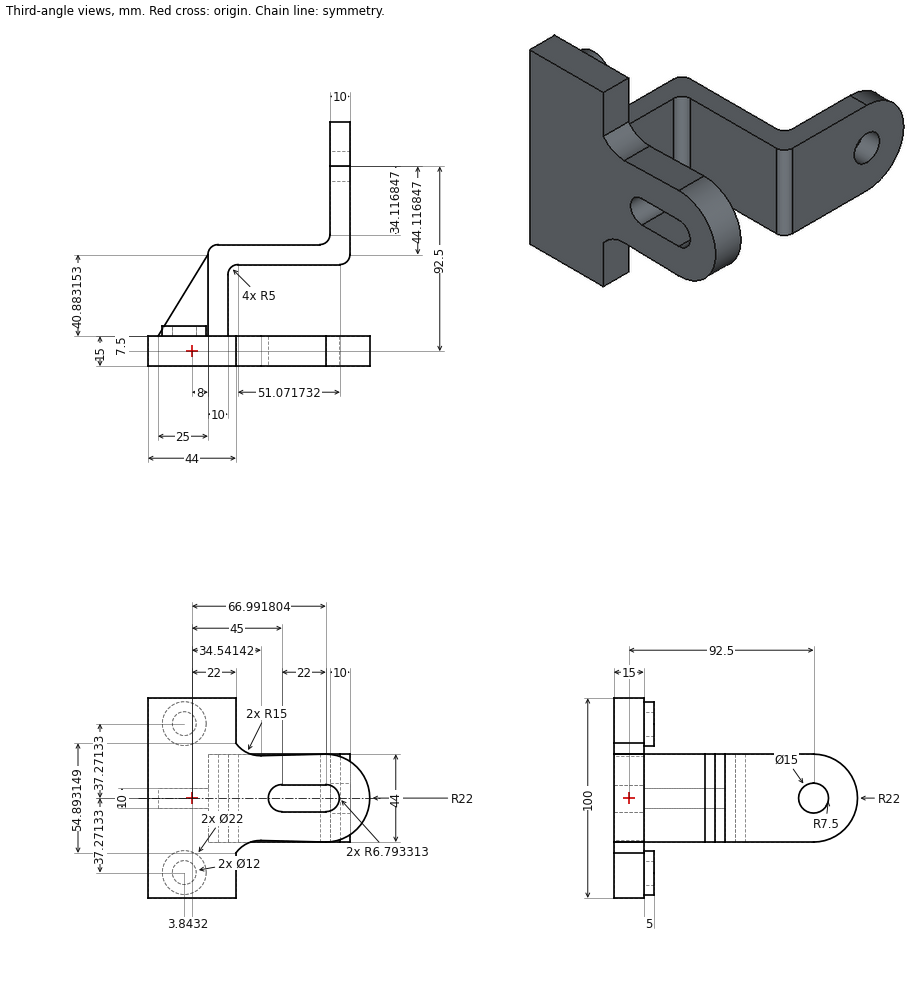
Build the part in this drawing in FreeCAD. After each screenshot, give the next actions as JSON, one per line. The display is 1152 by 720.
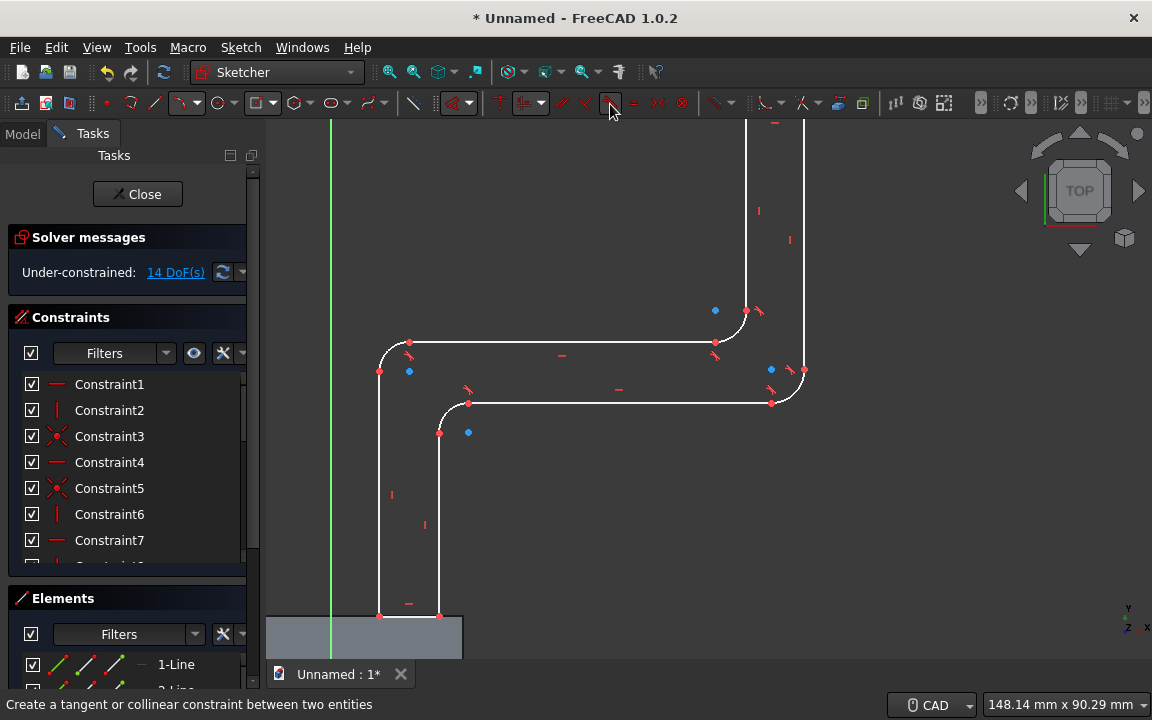
{"action": "left_click", "coordinate": [379, 445]}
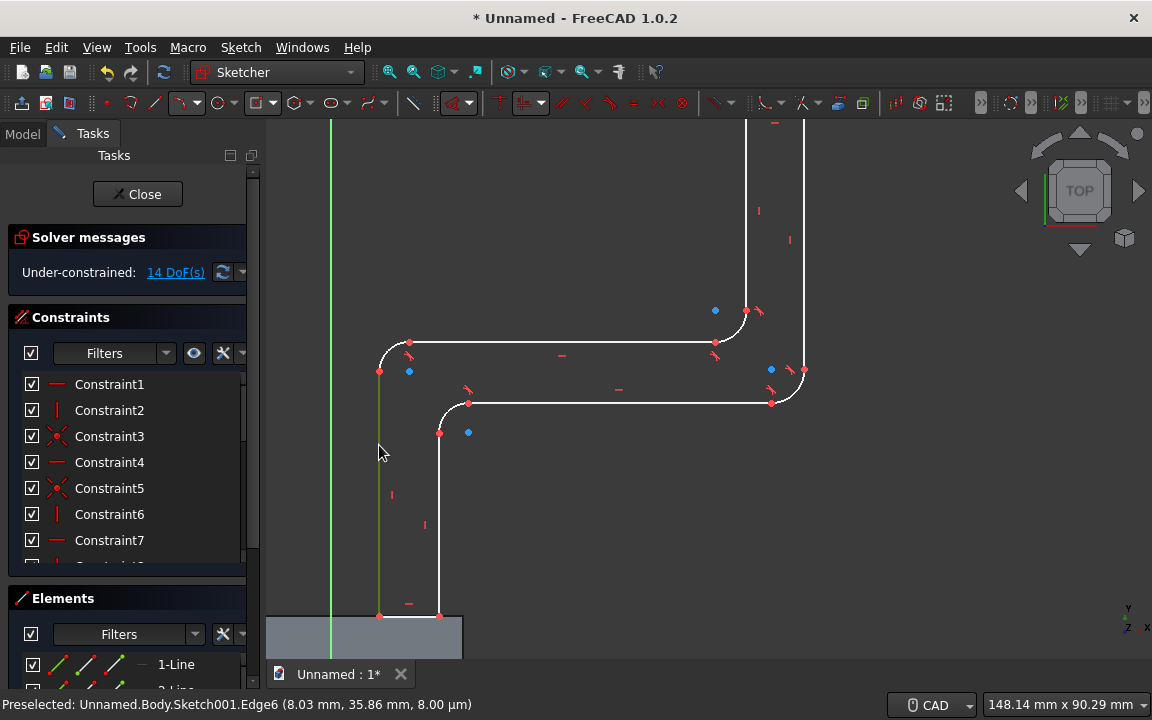
{"action": "left_click", "coordinate": [396, 345]}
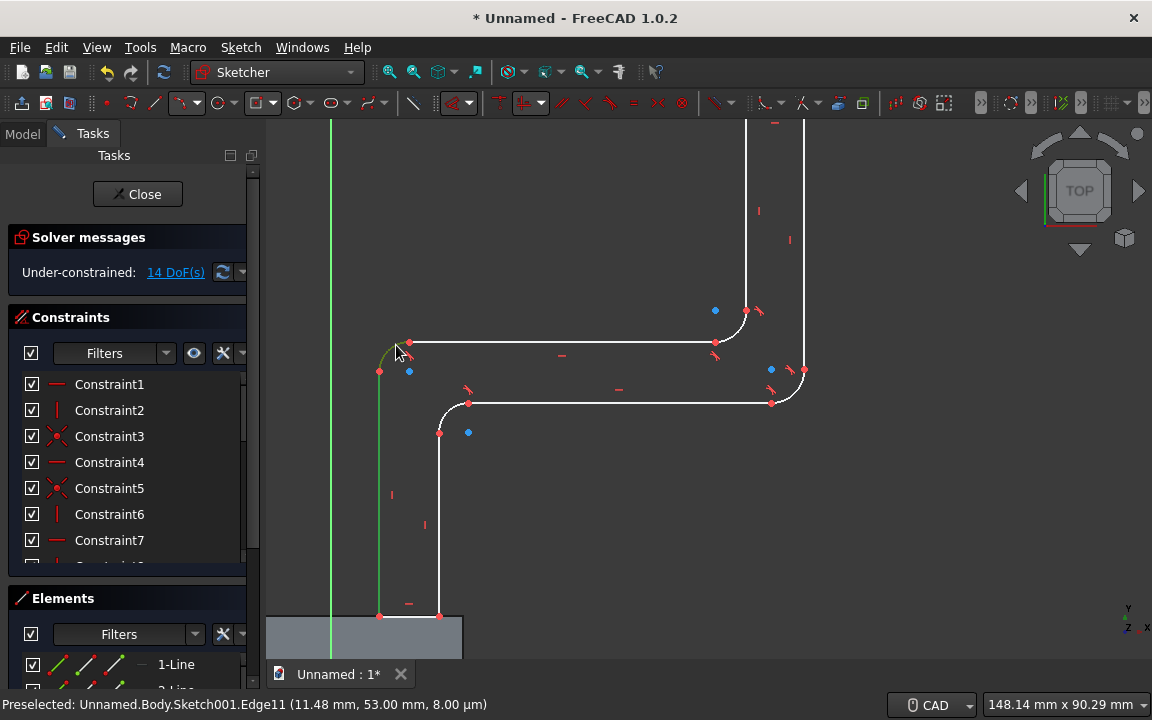
{"action": "left_click", "coordinate": [610, 104]}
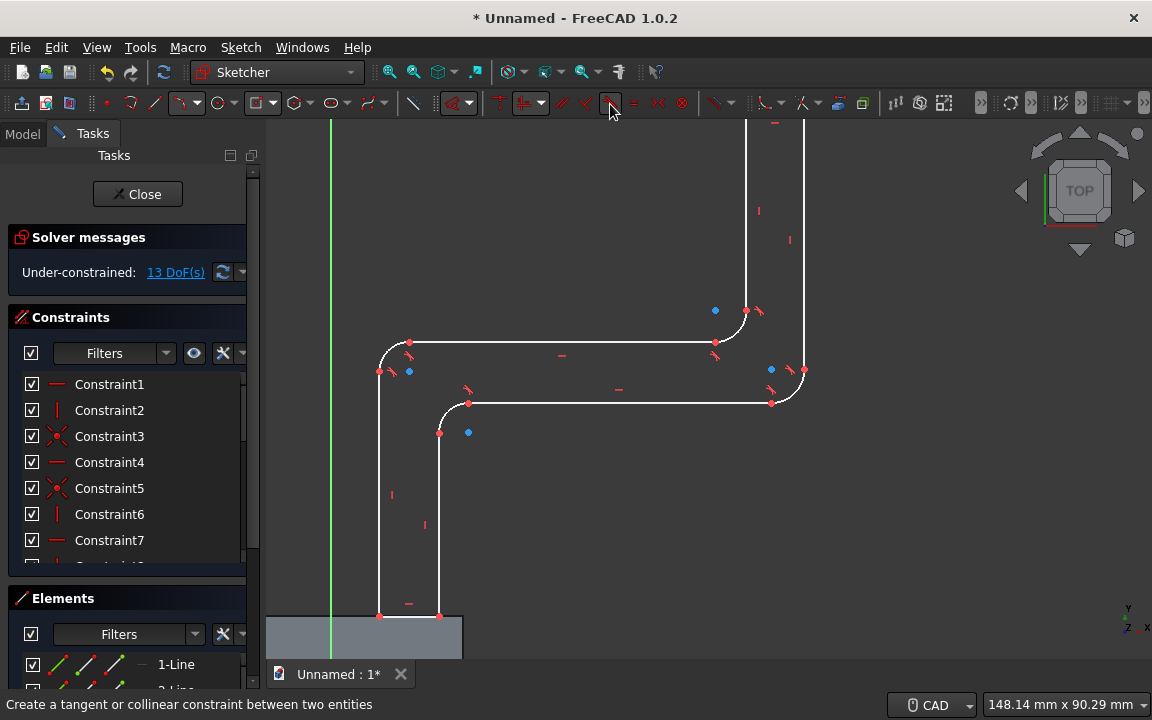
{"action": "left_click", "coordinate": [439, 562]}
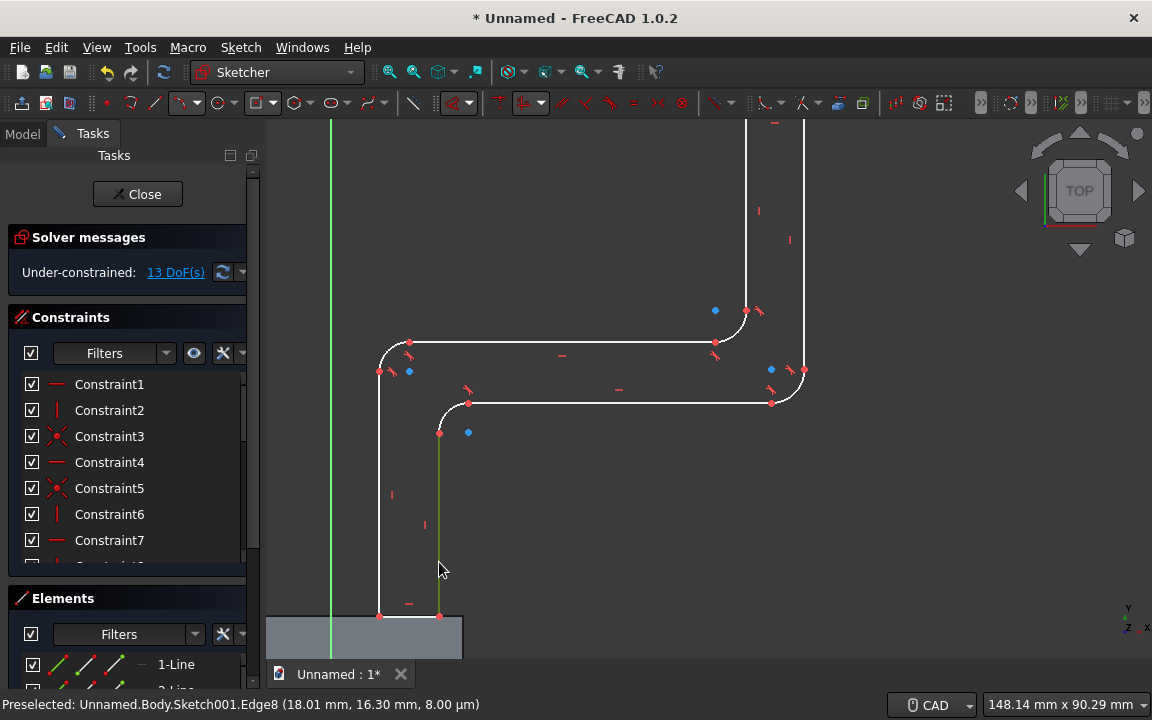
{"action": "left_click", "coordinate": [455, 406]}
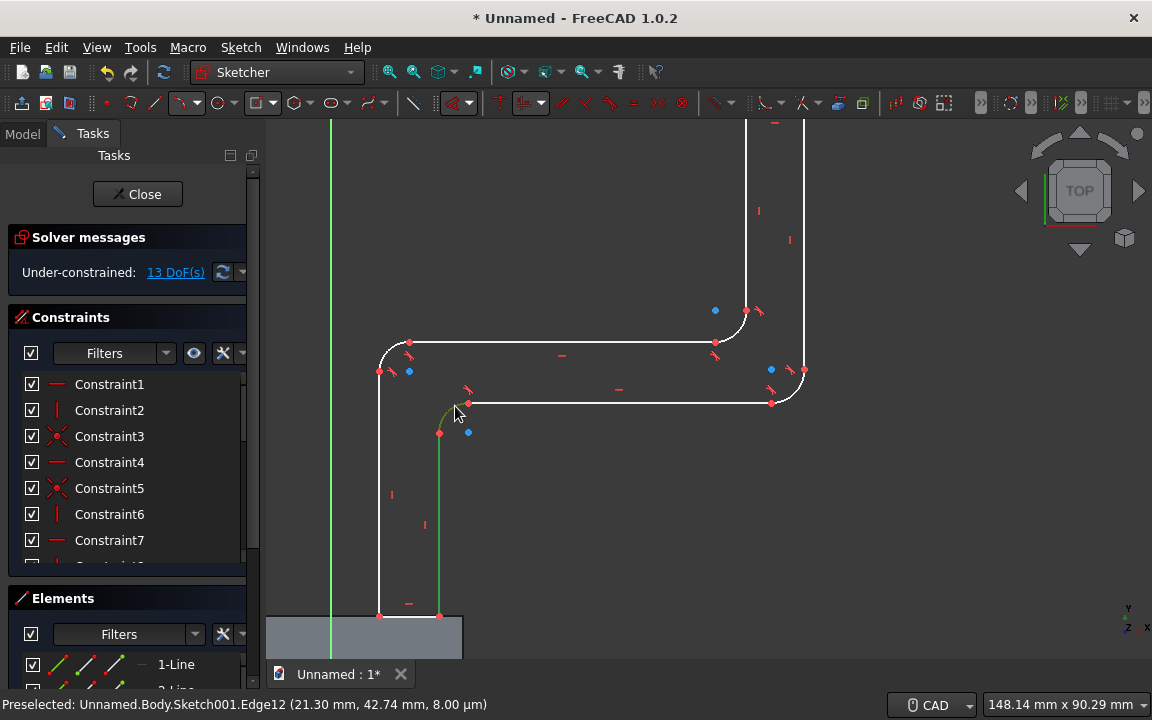
{"action": "left_click", "coordinate": [610, 104]}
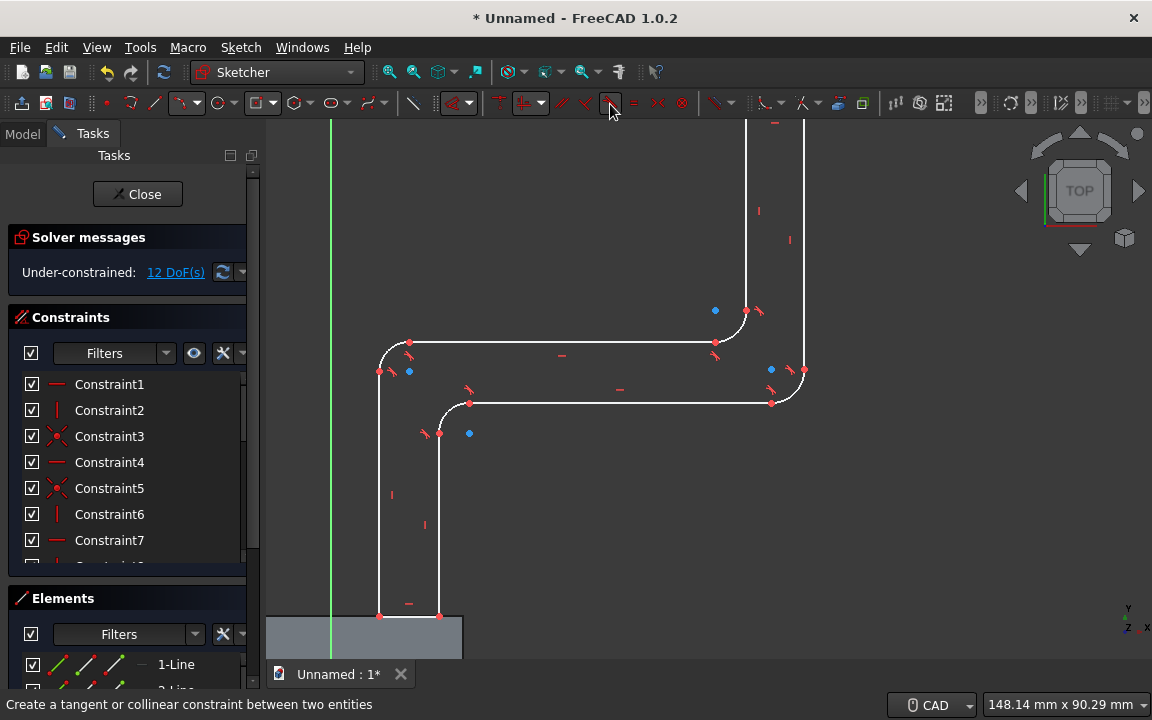
{"action": "left_click", "coordinate": [786, 399]}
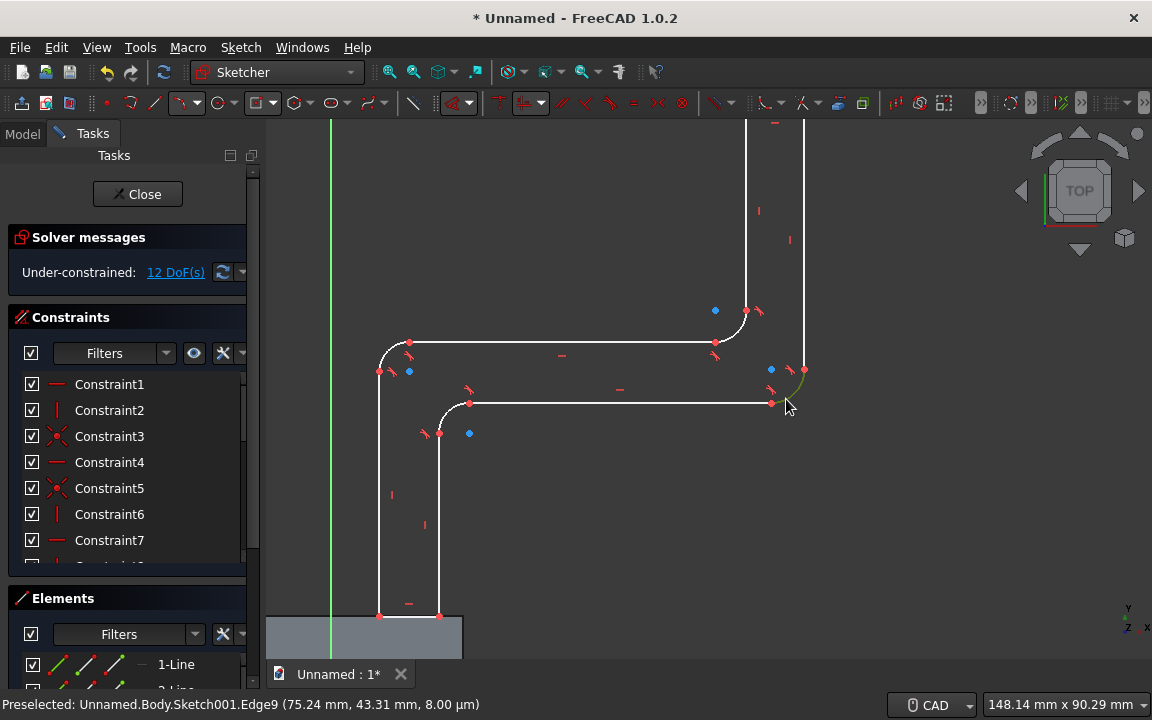
{"action": "left_click", "coordinate": [729, 339]}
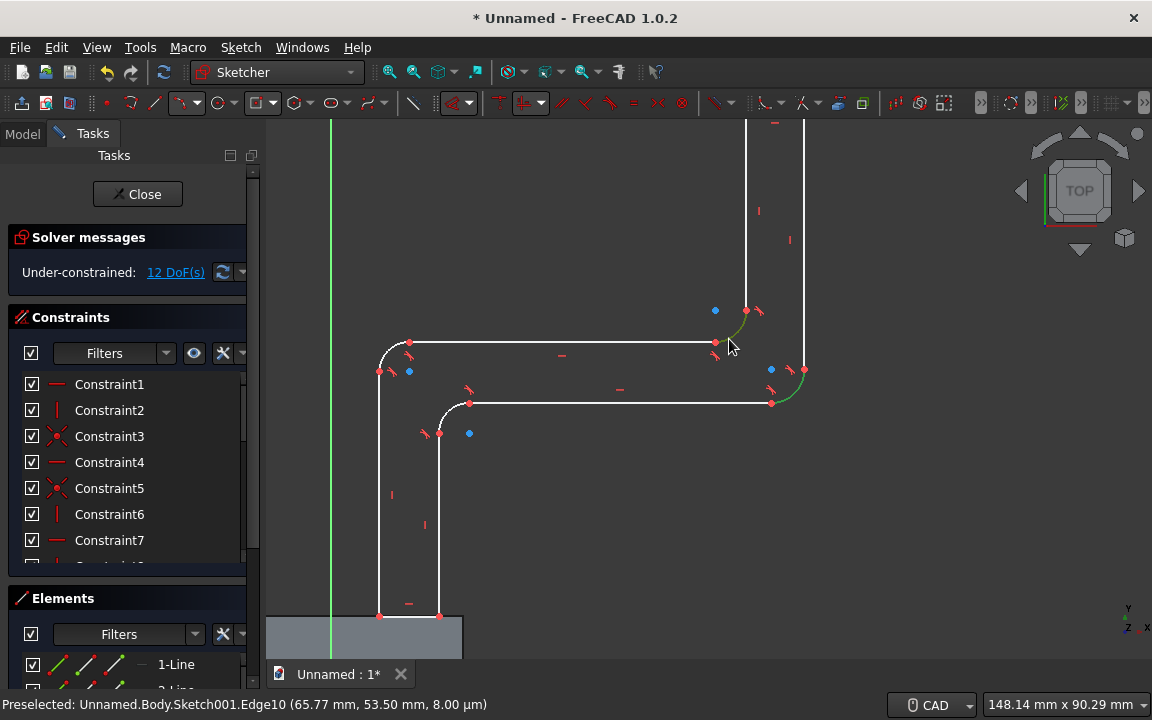
{"action": "left_click", "coordinate": [396, 345]}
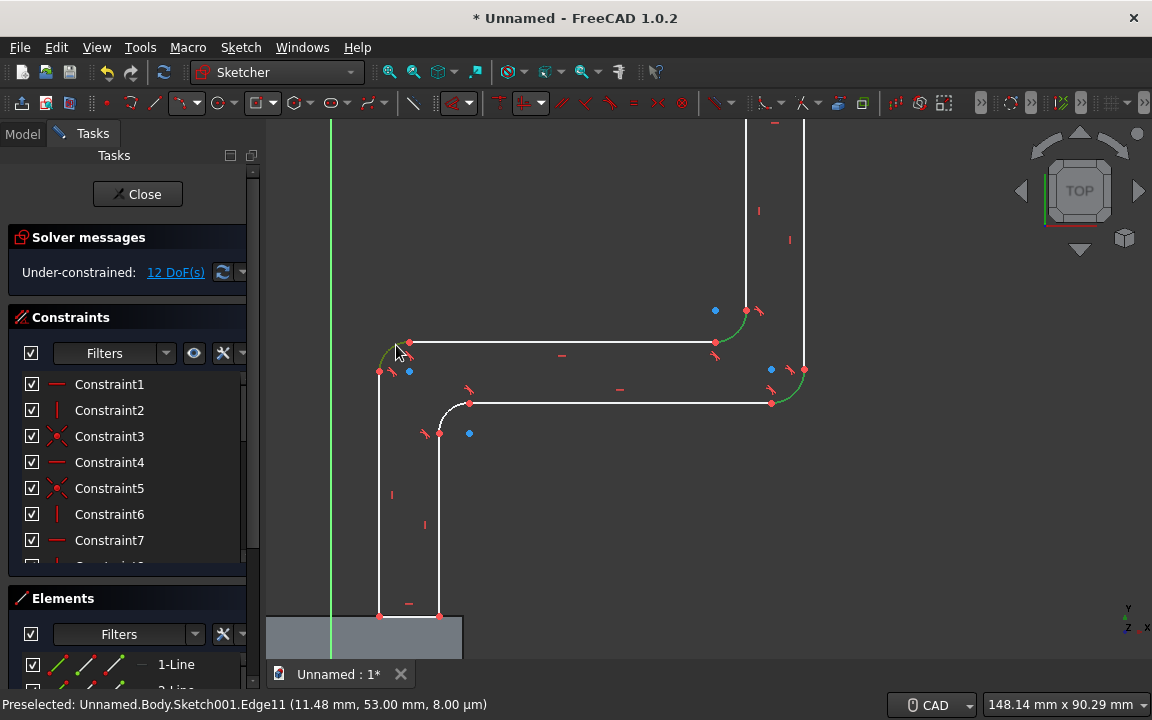
{"action": "left_click", "coordinate": [455, 406]}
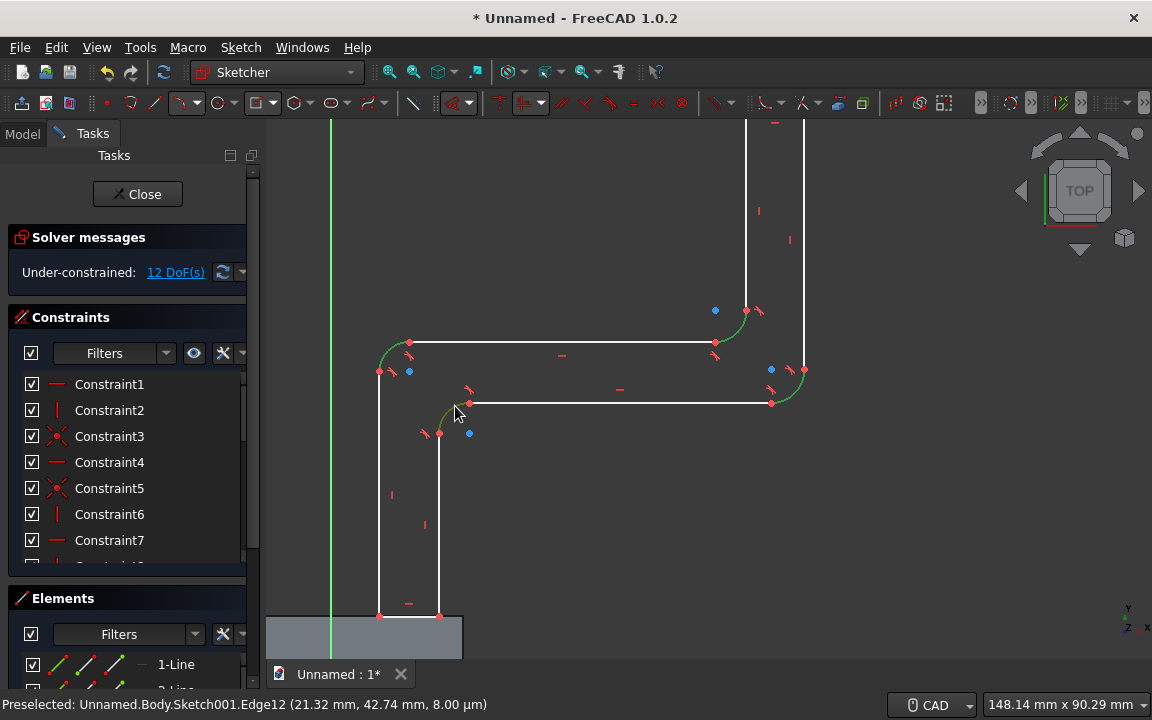
{"action": "left_click", "coordinate": [634, 104]}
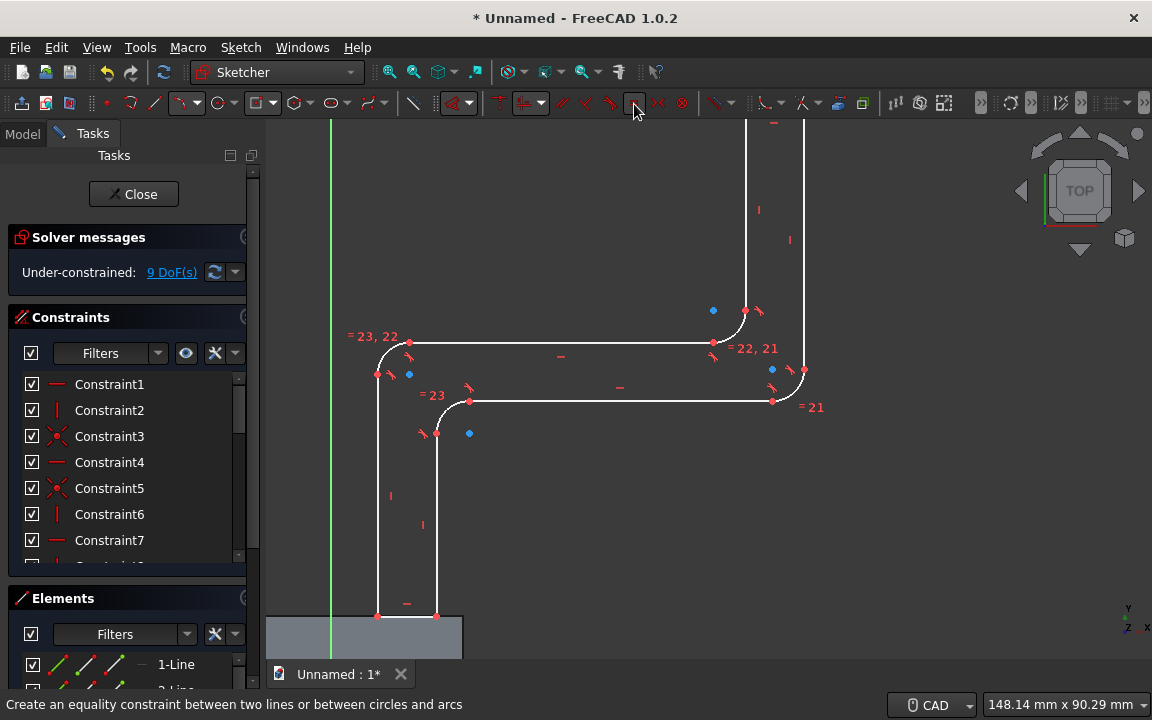
{"action": "left_click", "coordinate": [452, 104]}